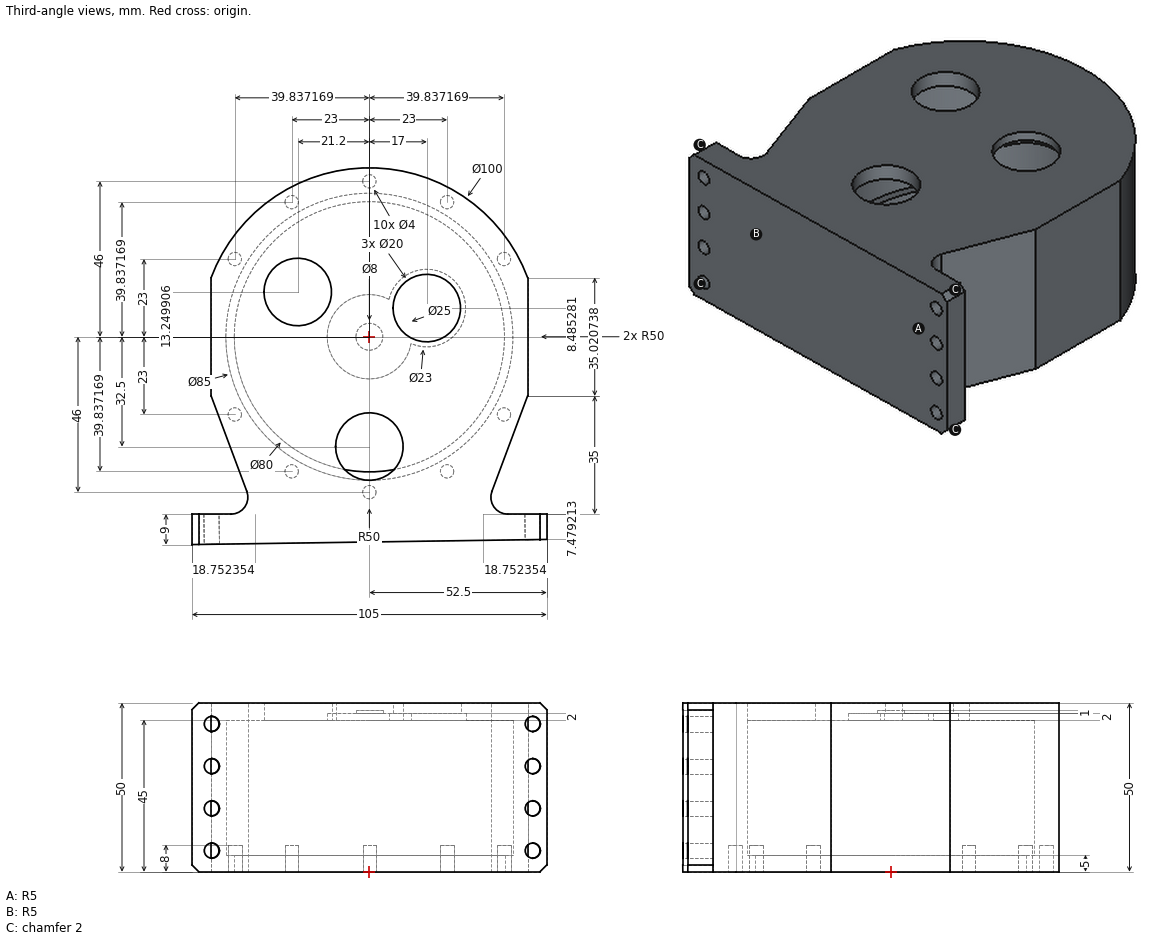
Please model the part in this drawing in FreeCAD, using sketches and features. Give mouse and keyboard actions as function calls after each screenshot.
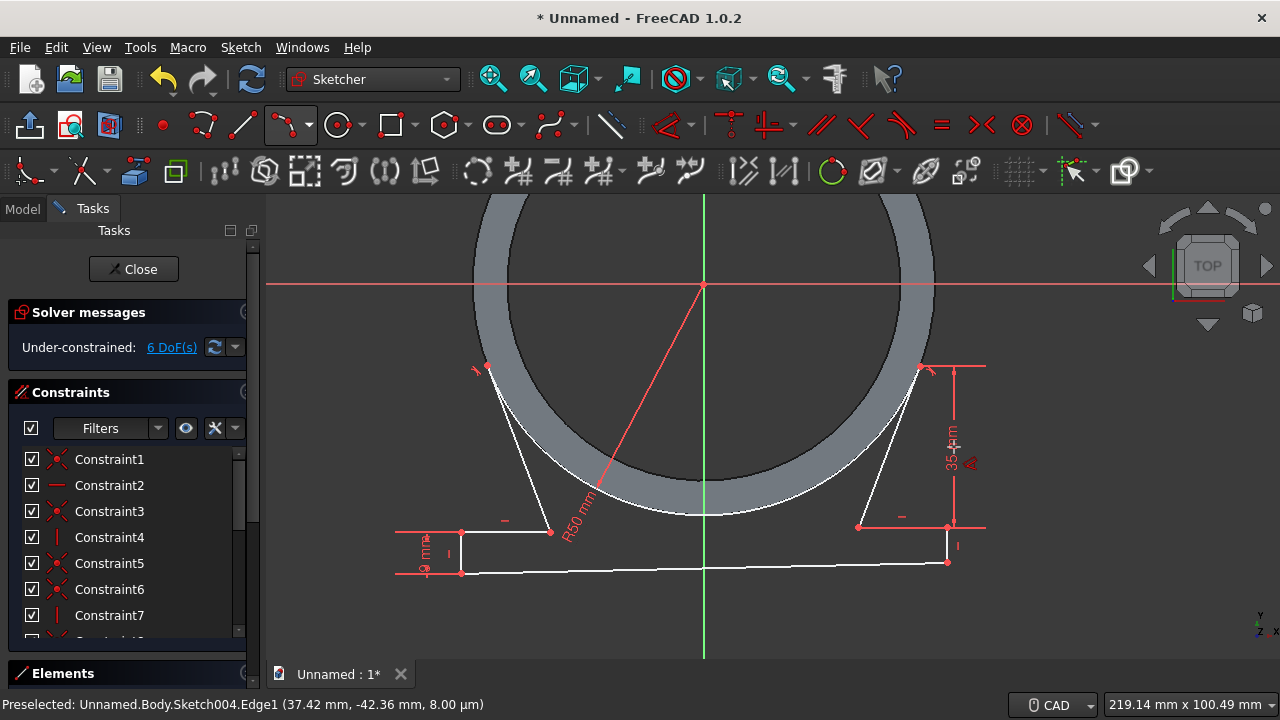
click(532, 482)
click(454, 449)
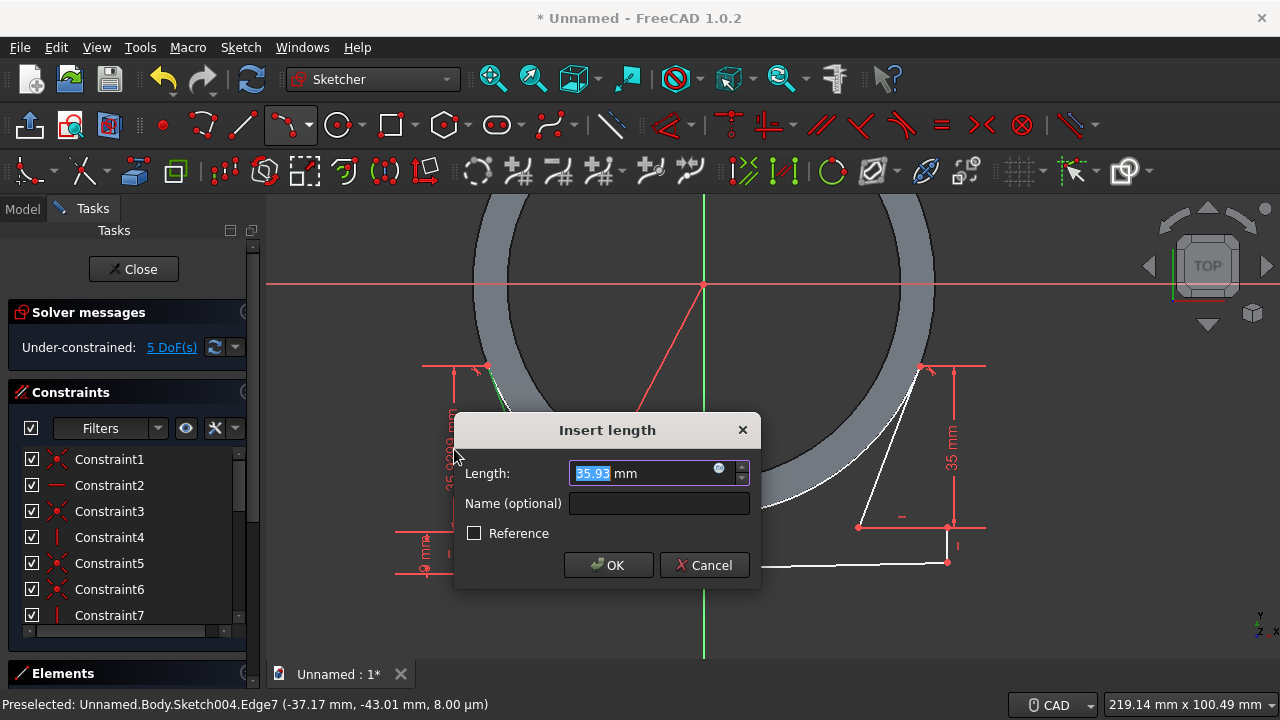
text(35)
key(Return)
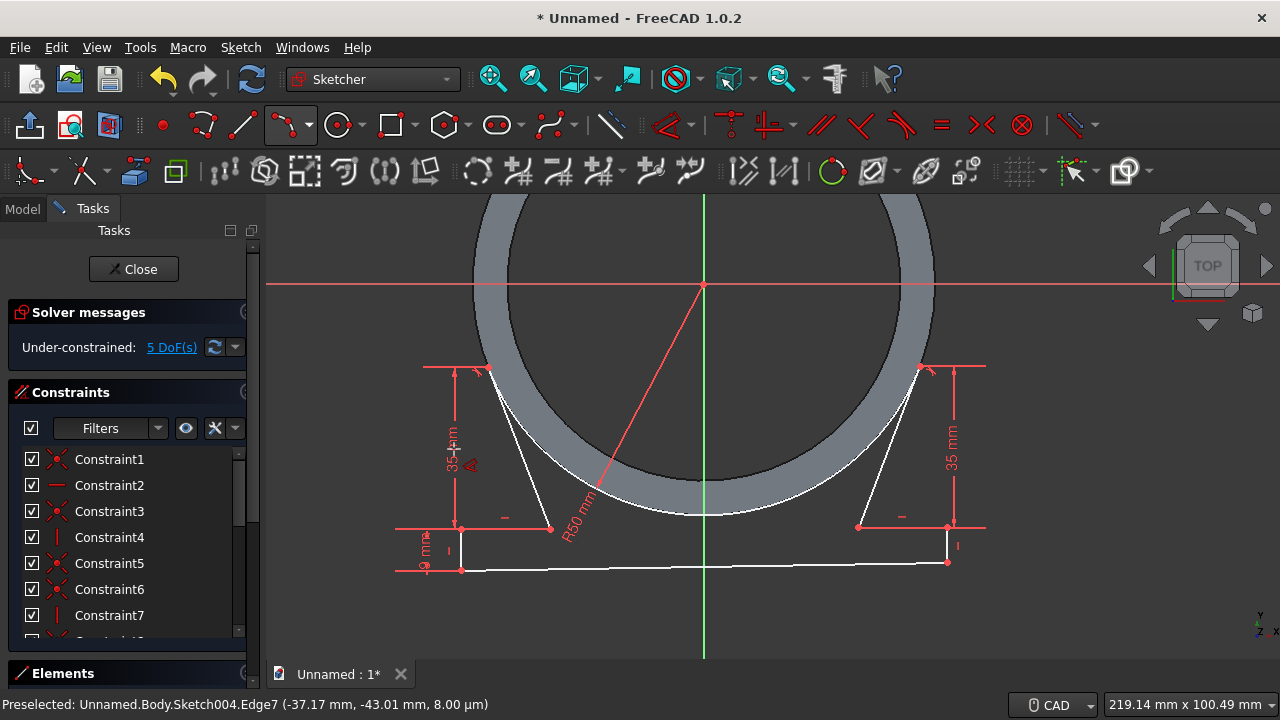
click(801, 565)
click(592, 605)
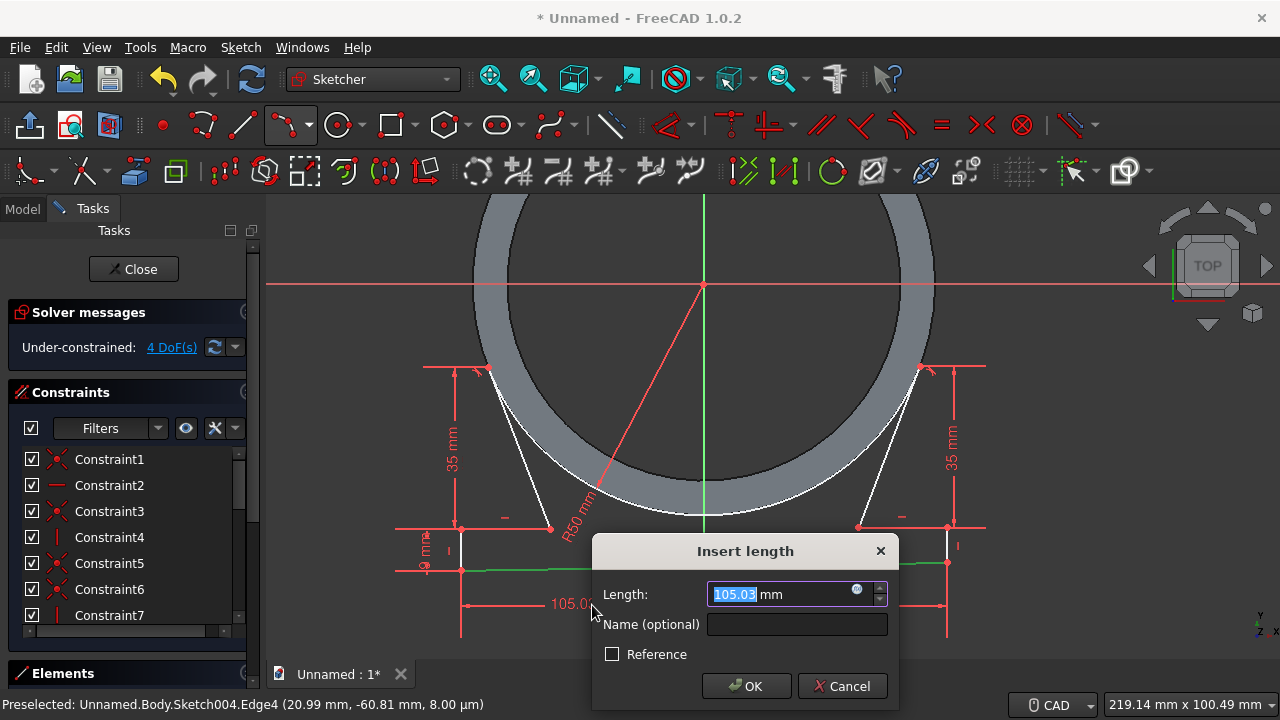
text(105)
key(Return)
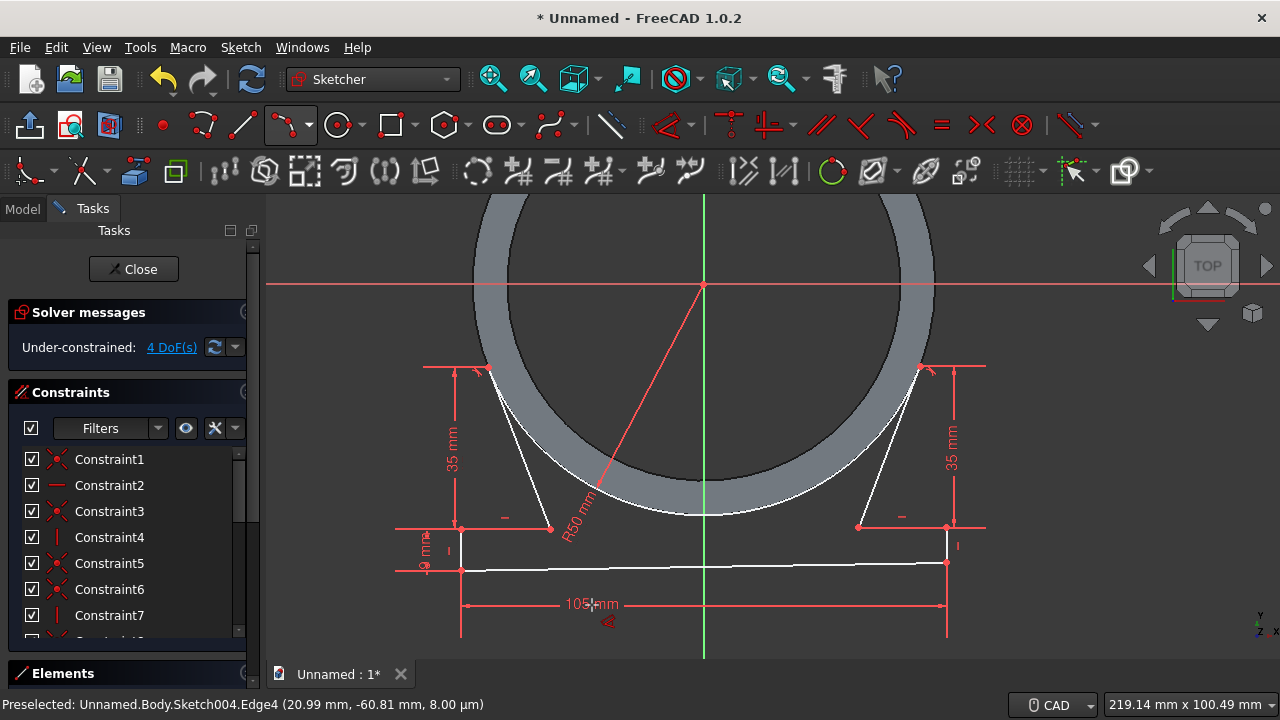
click(947, 528)
click(825, 250)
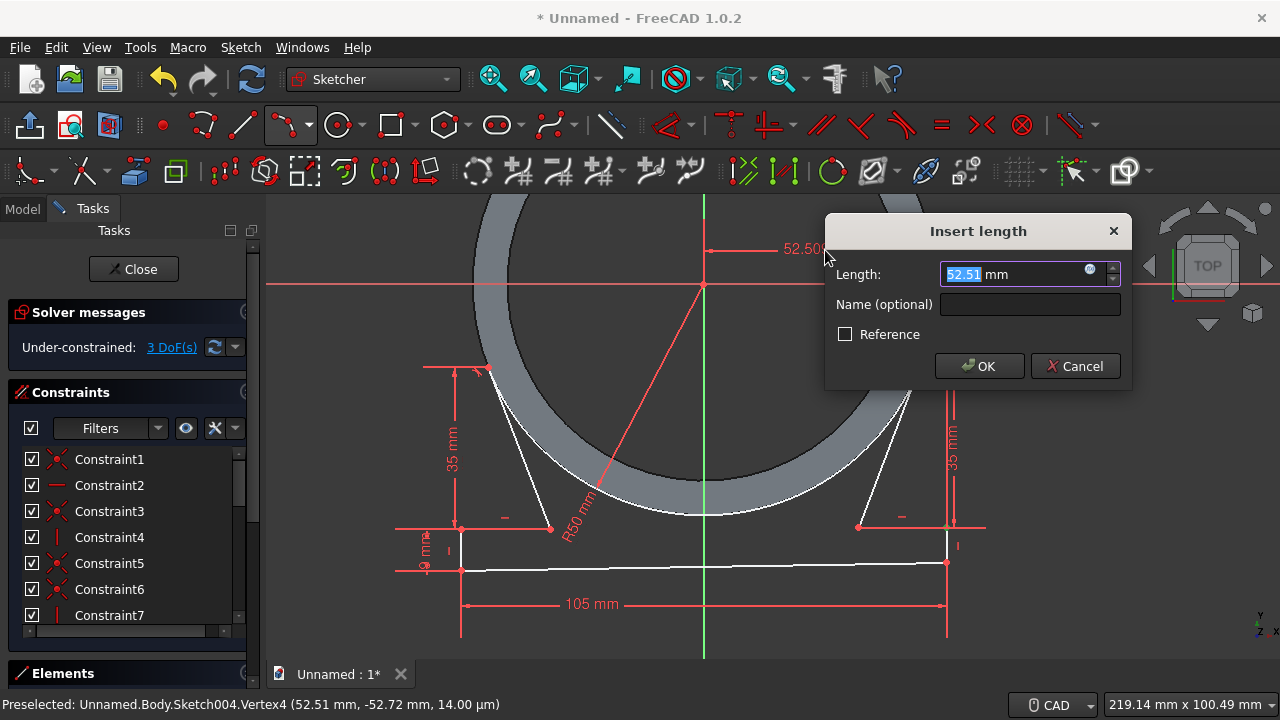
text(52.5)
key(Return)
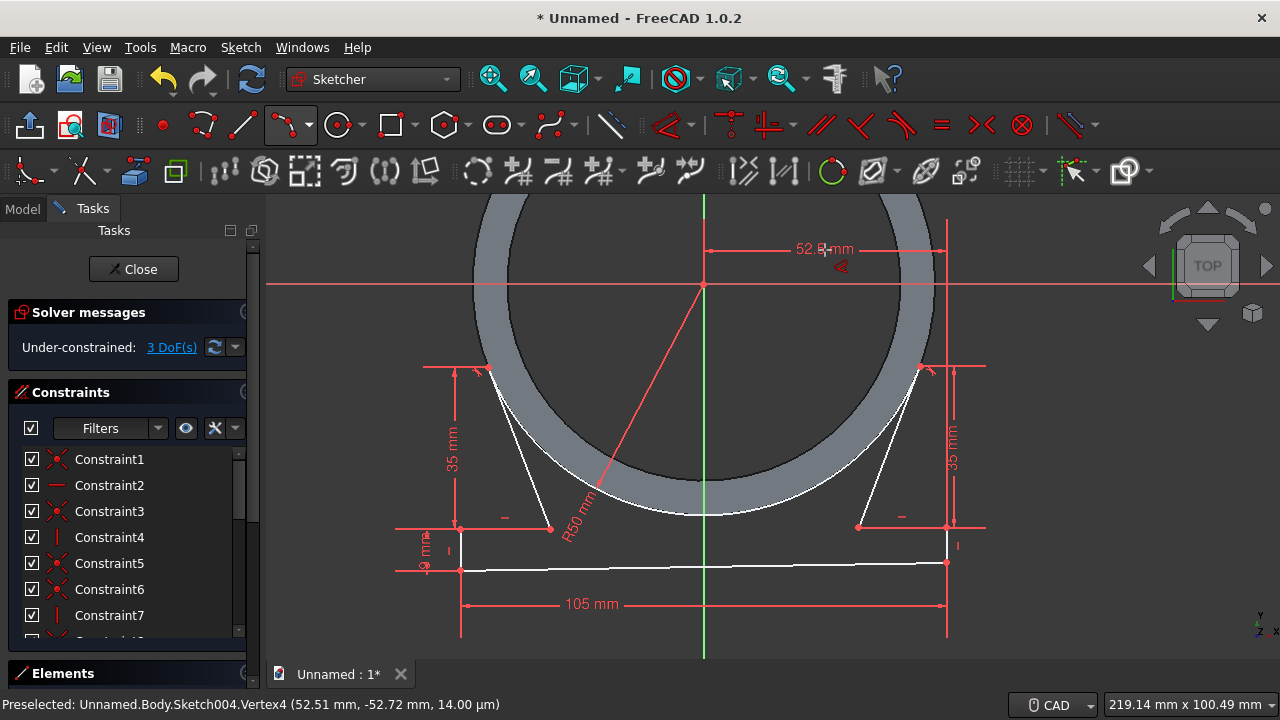
scroll(947, 538, up, 2)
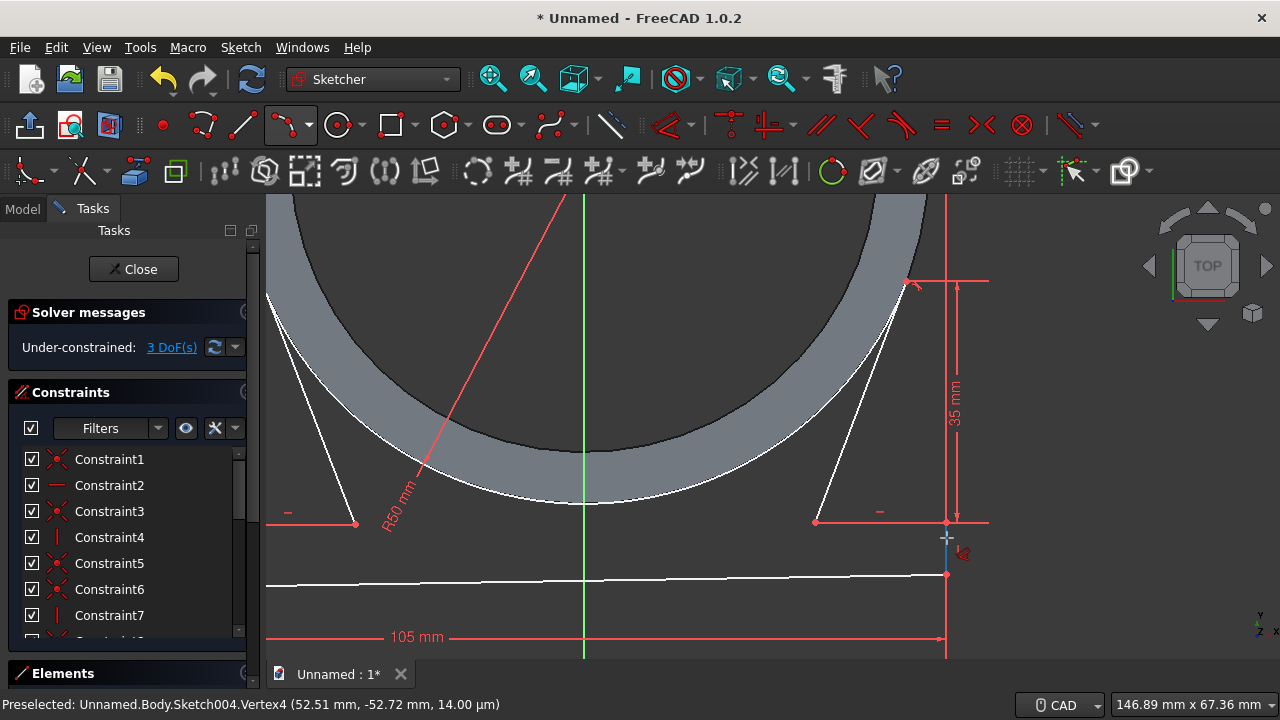
click(946, 538)
click(980, 549)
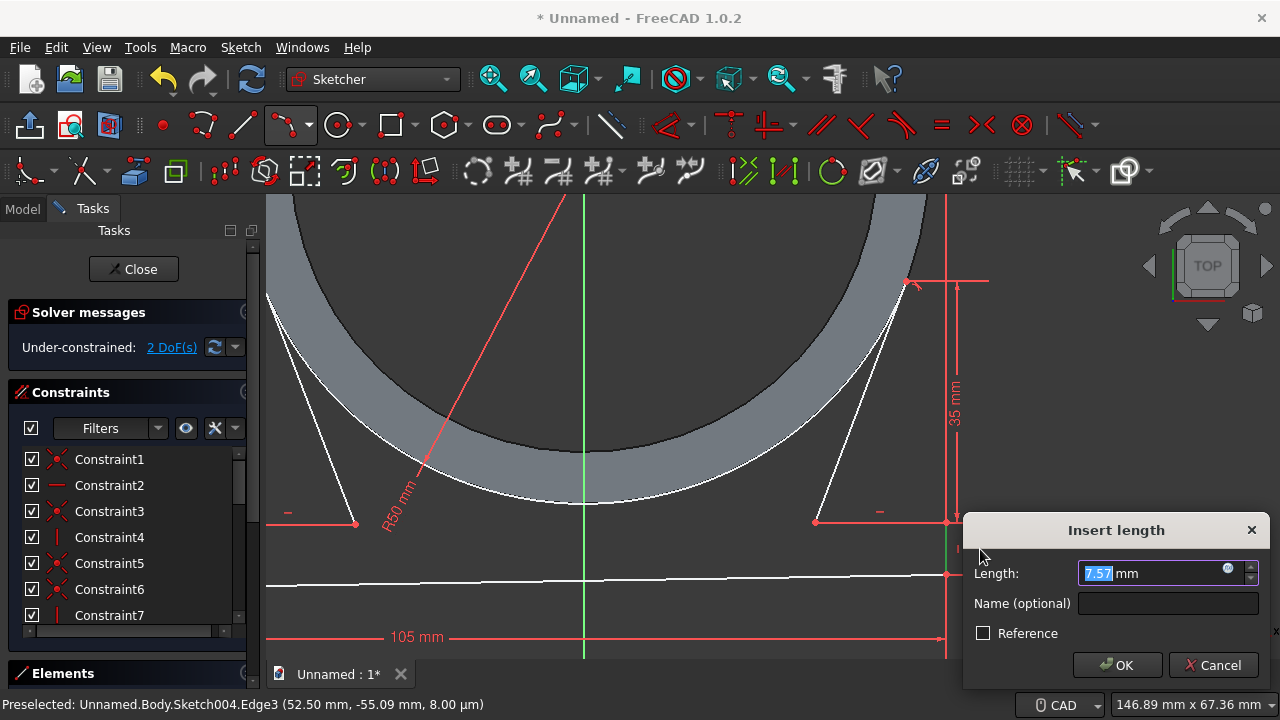
text(7.479213)
key(Return)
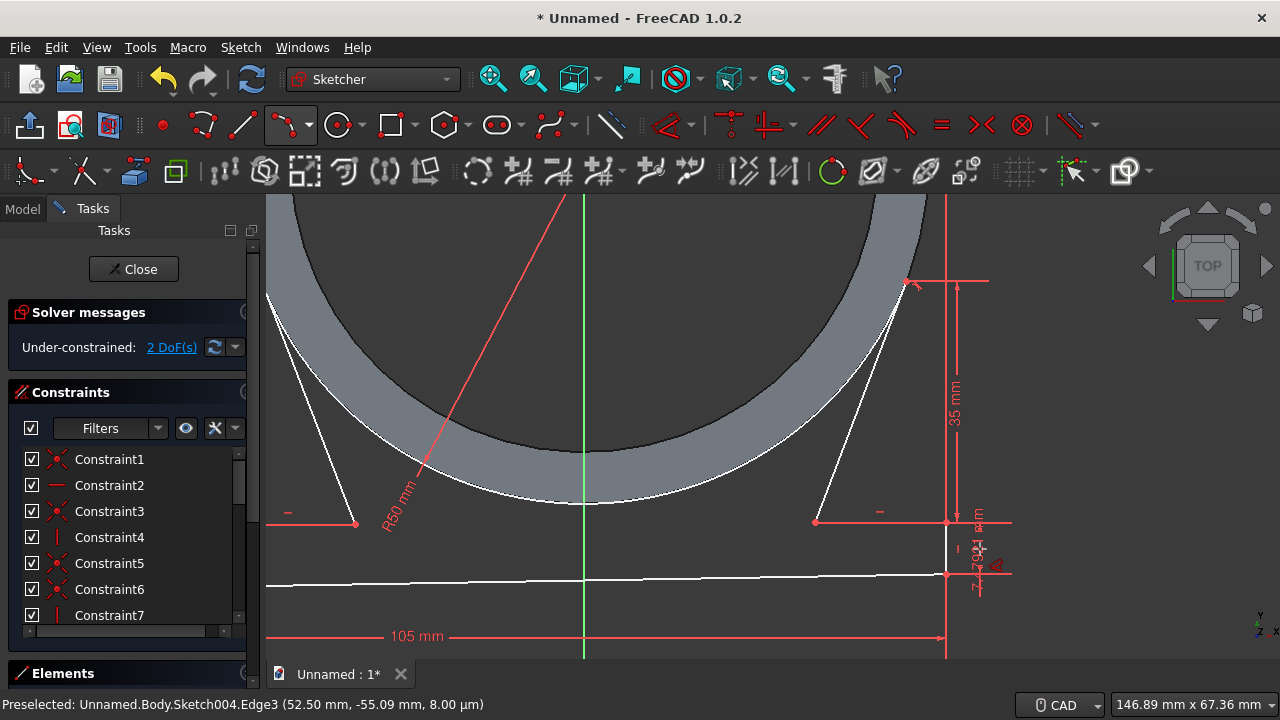
click(854, 523)
click(881, 557)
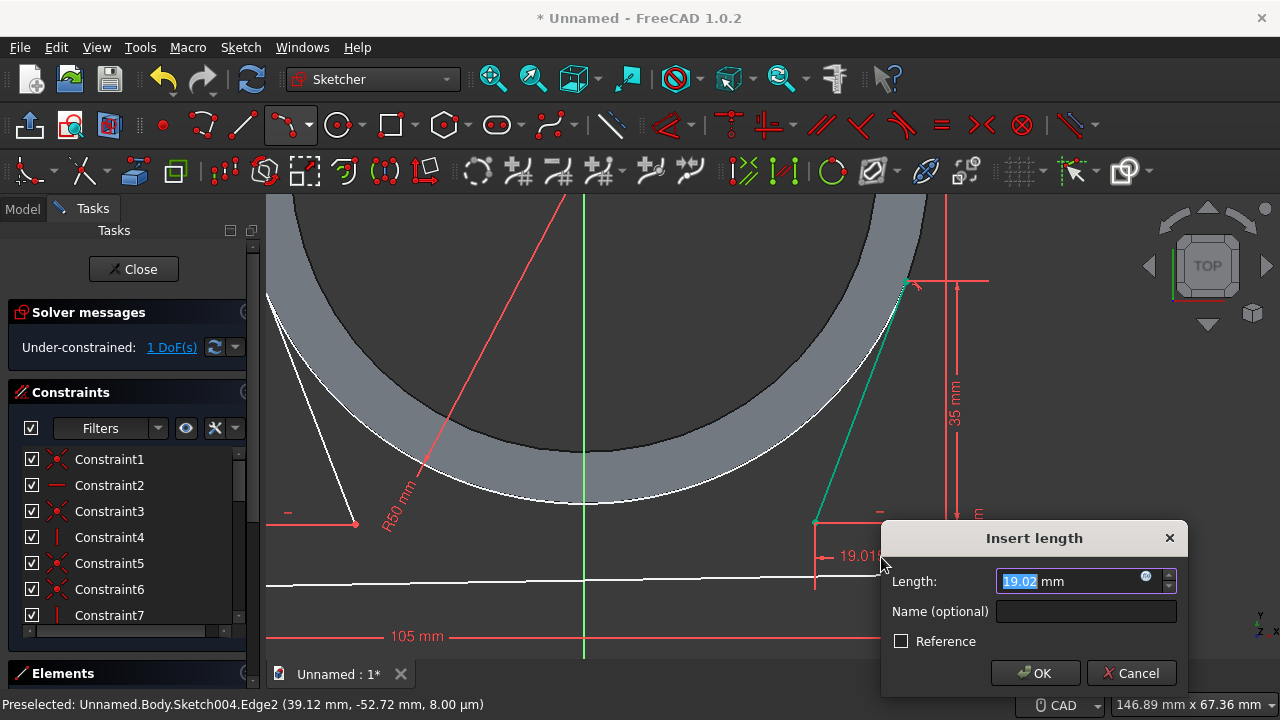
text(18.752354)
key(Return)